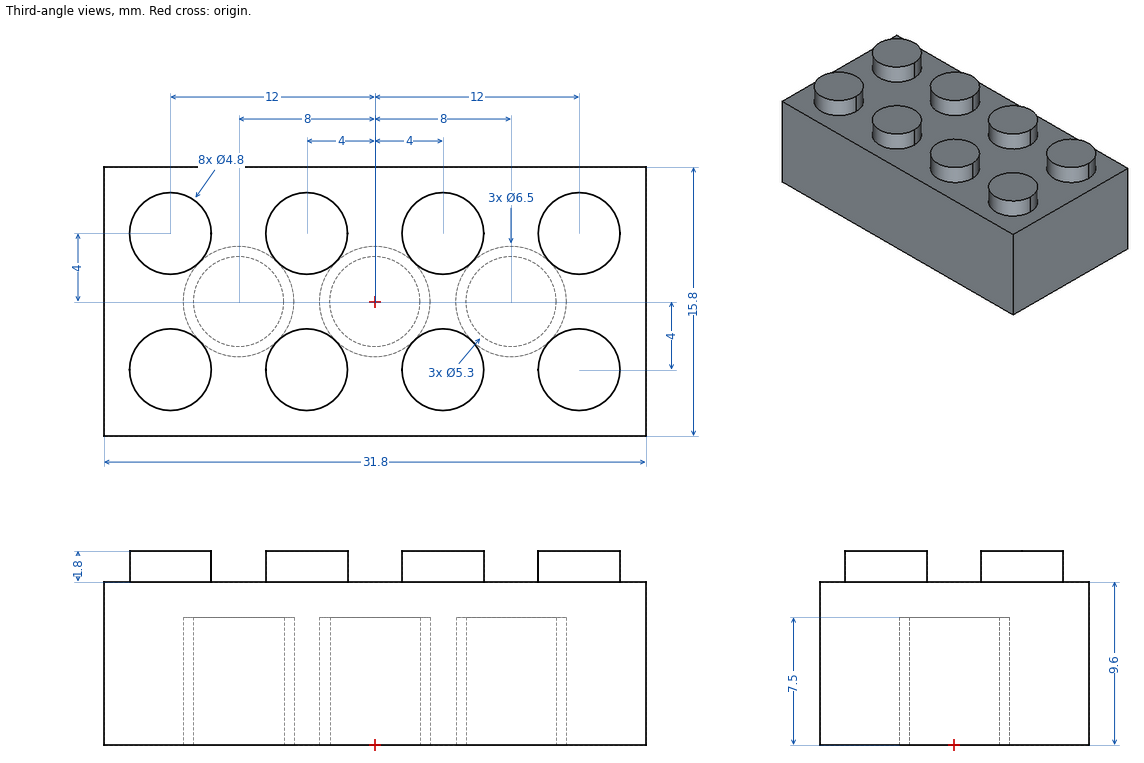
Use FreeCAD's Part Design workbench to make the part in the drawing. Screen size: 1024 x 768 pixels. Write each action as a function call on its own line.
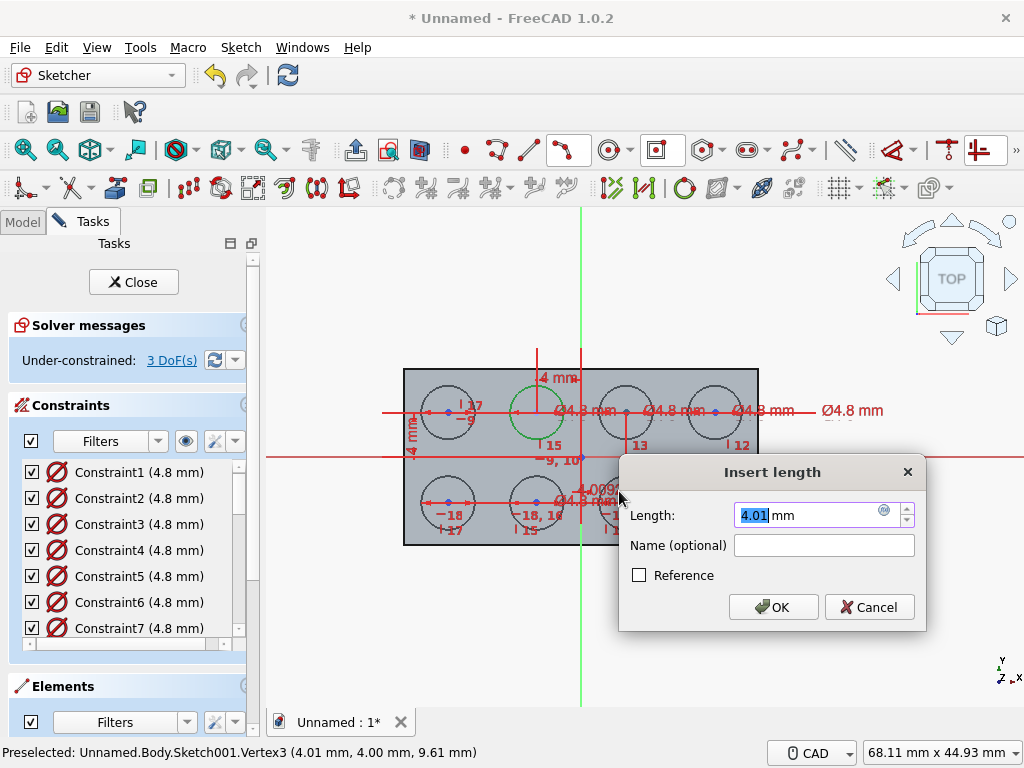
text(4)
key(Return)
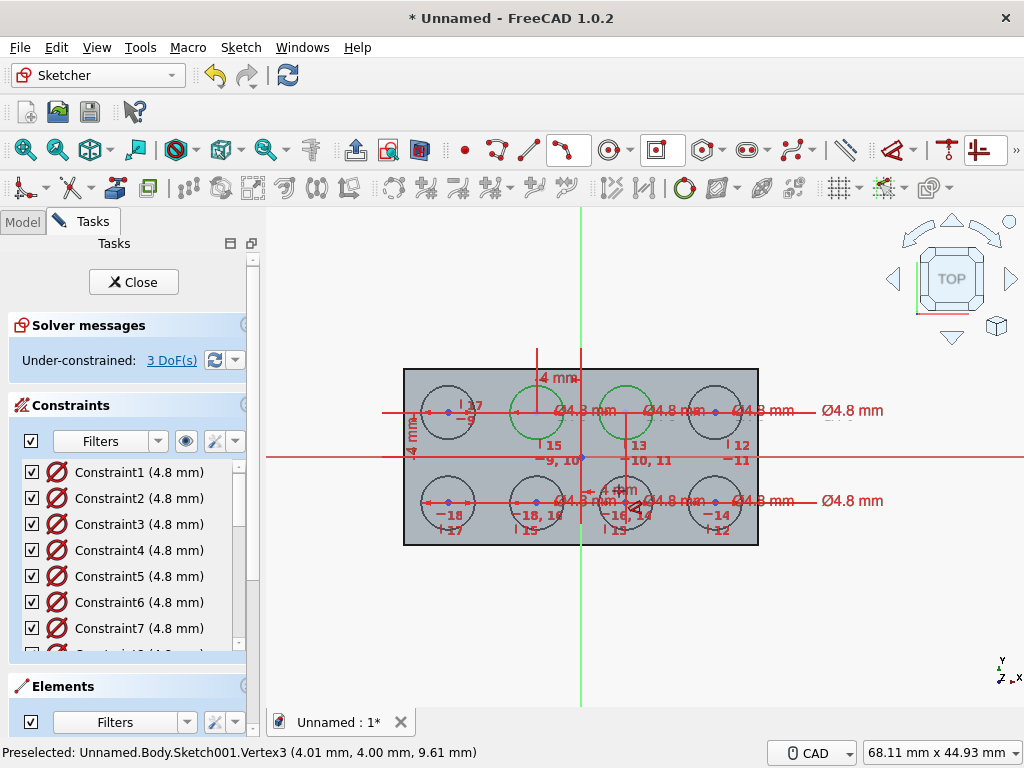
click(715, 503)
click(749, 480)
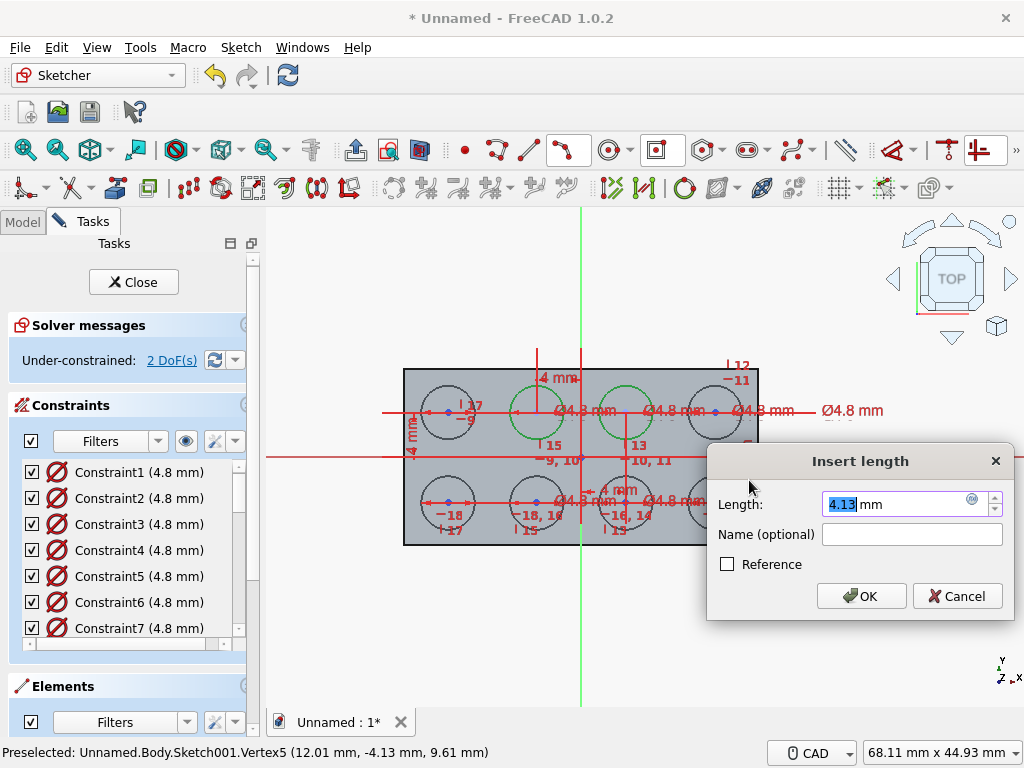
text(4)
key(Return)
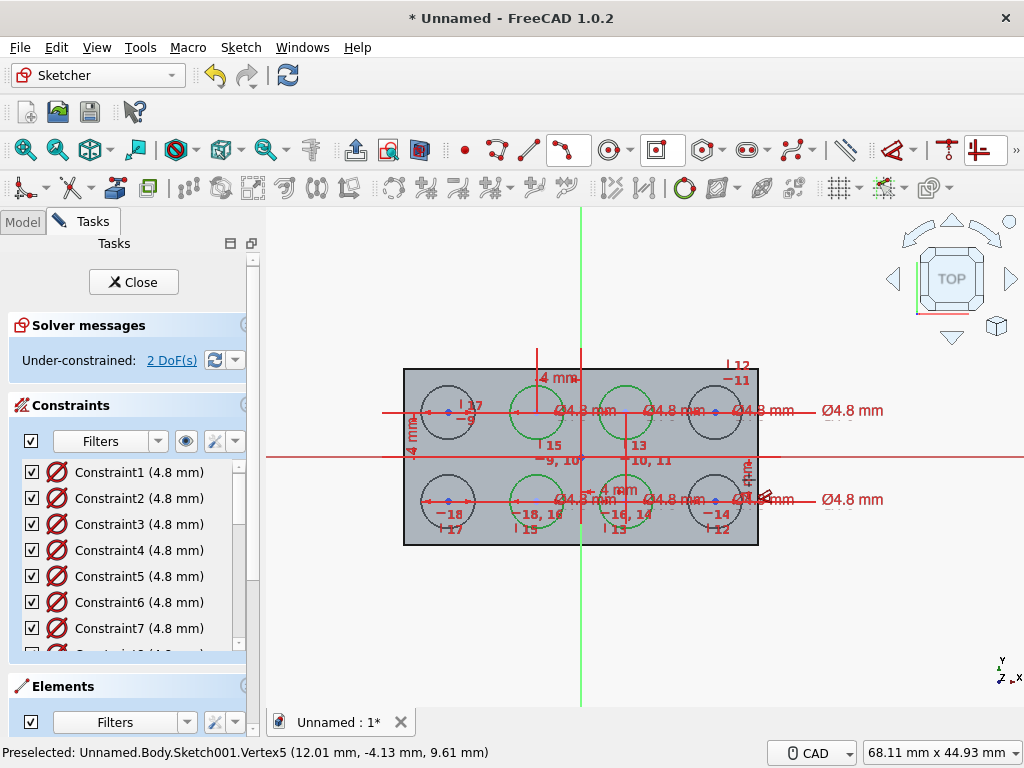
click(448, 413)
click(484, 379)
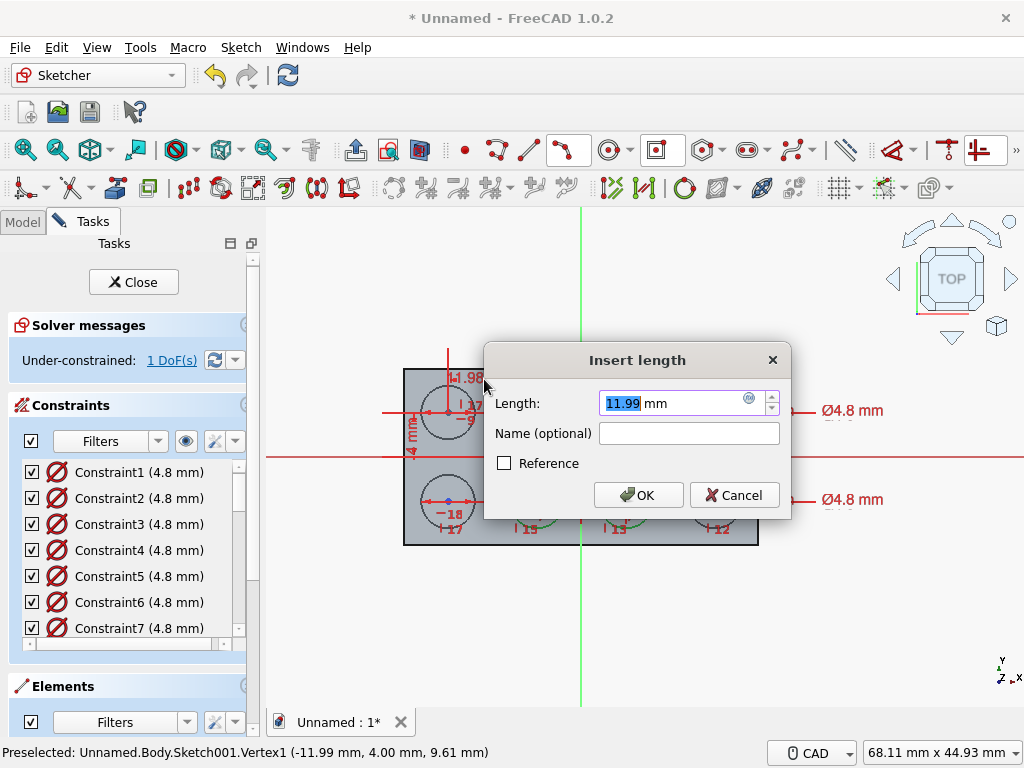
text(12)
key(Return)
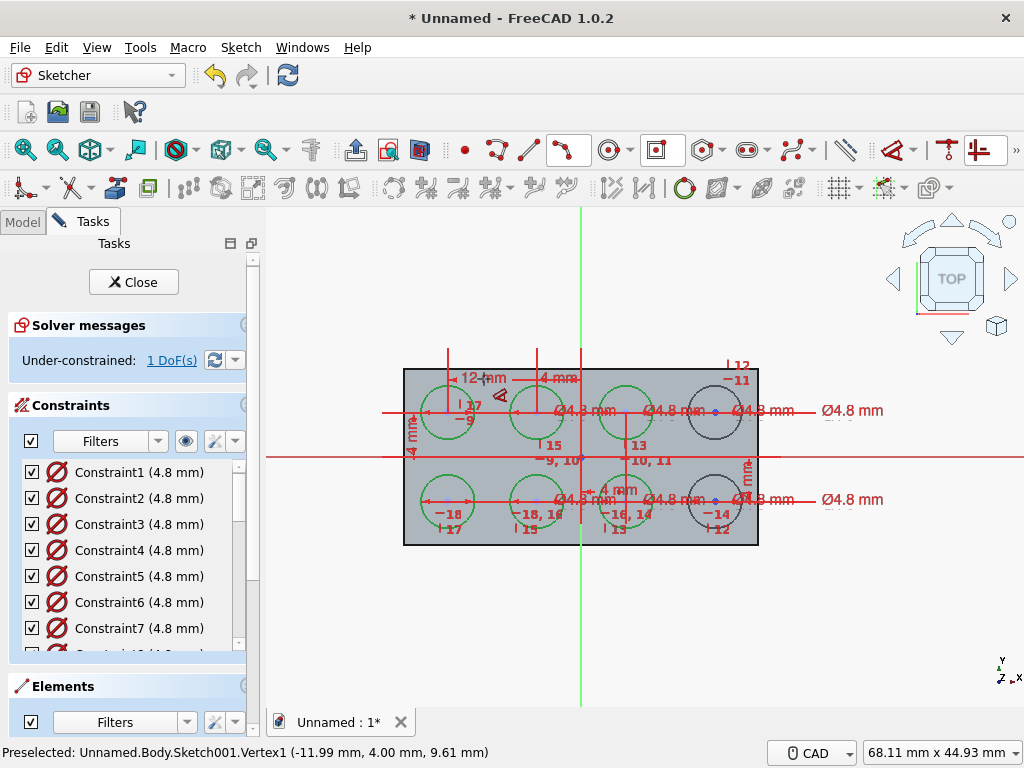
click(715, 413)
click(648, 379)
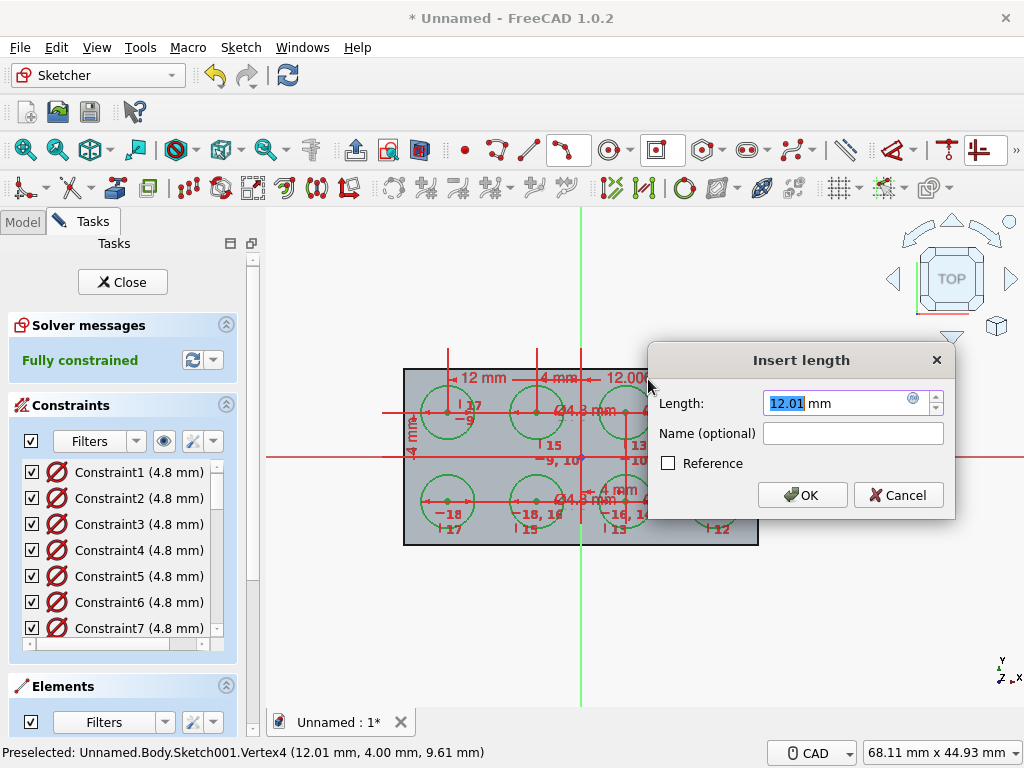
text(12)
key(Return)
key(Escape)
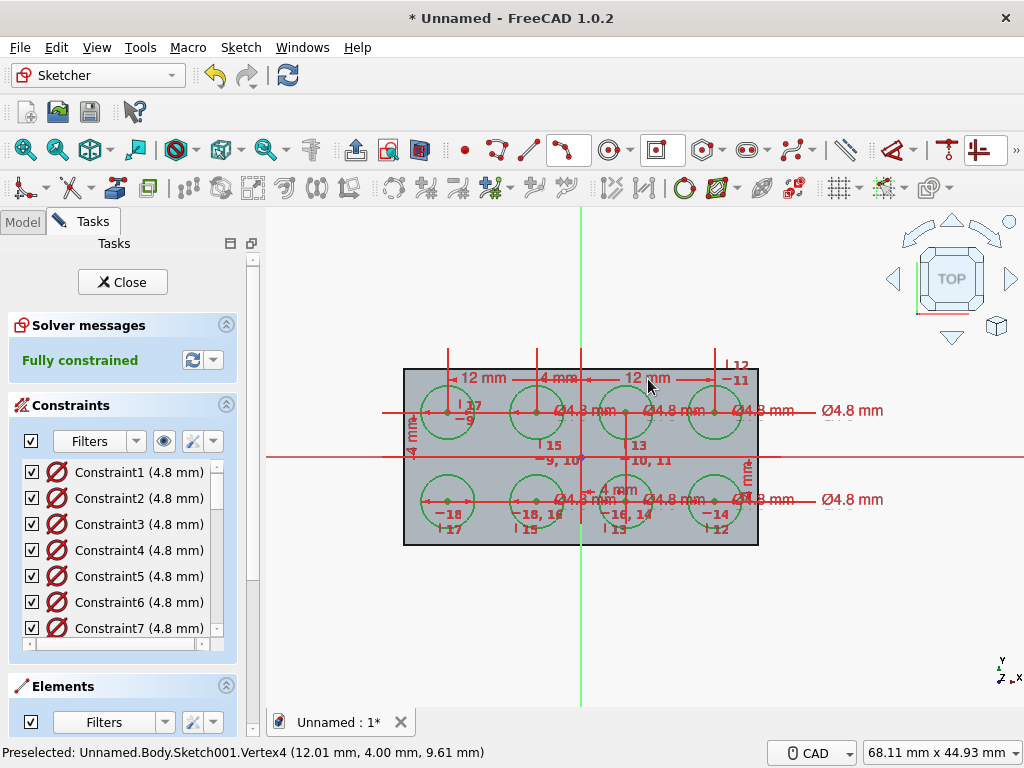
click(123, 282)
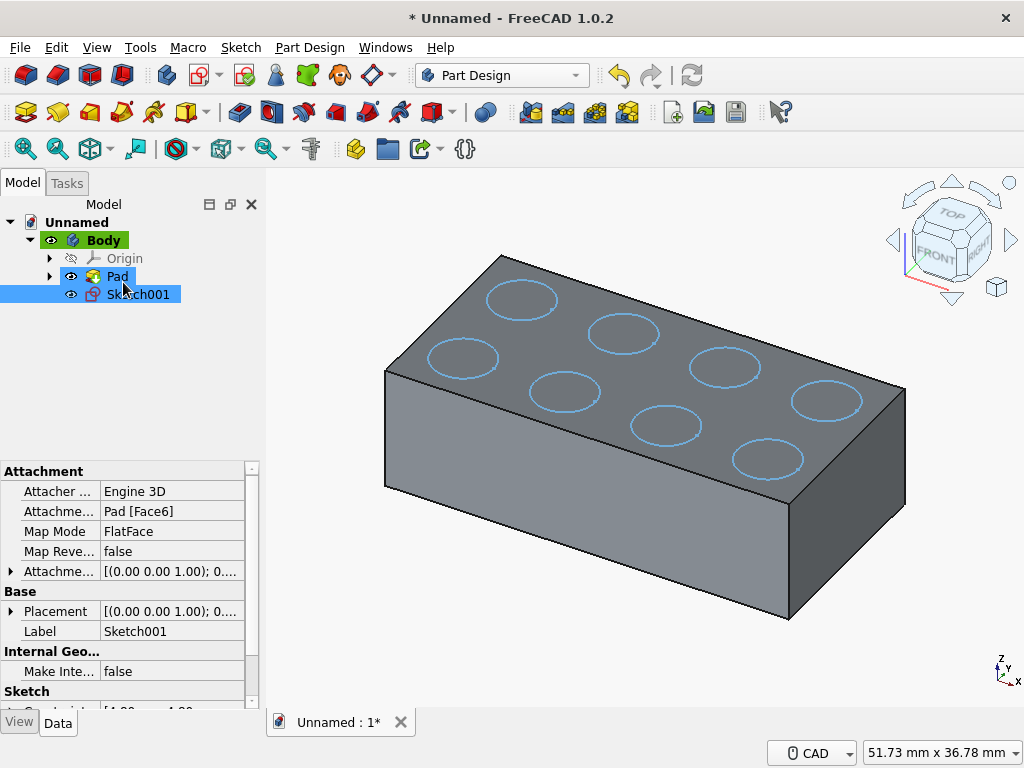
click(26, 112)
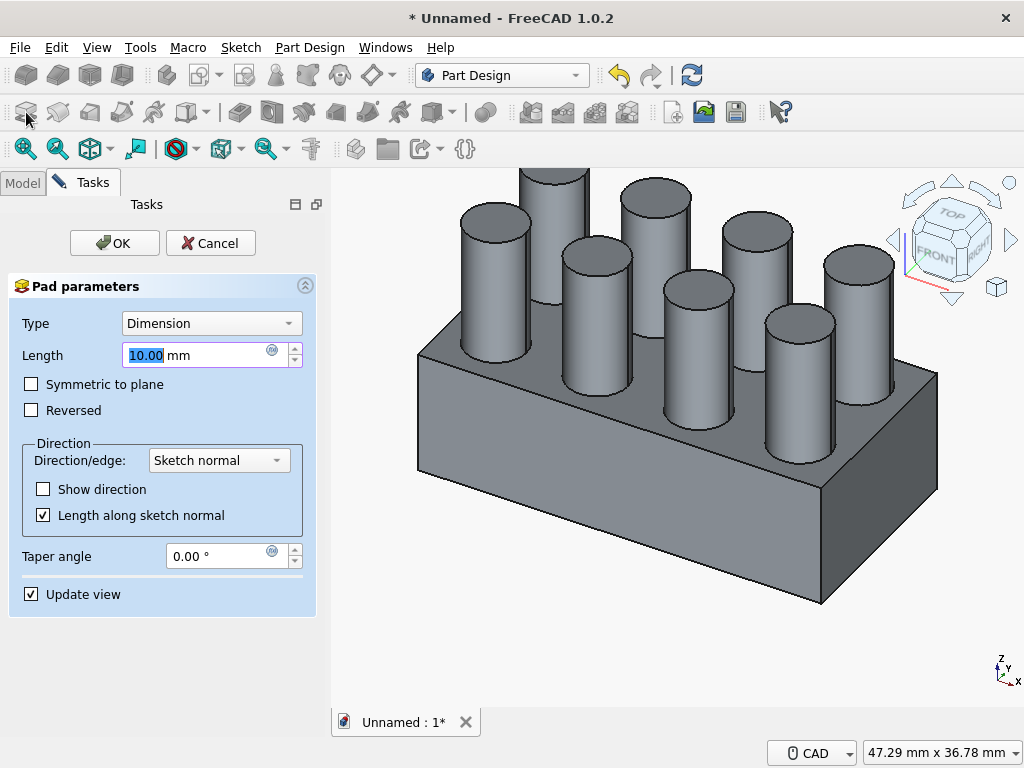
text(1.8)
key(Tab)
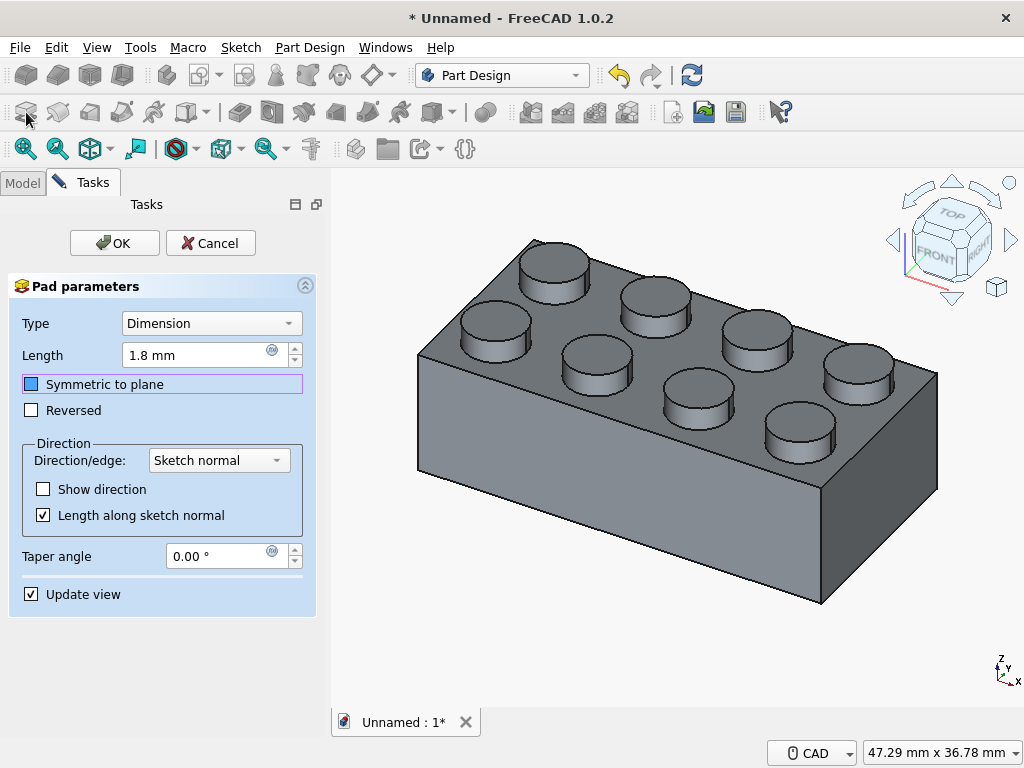
click(115, 243)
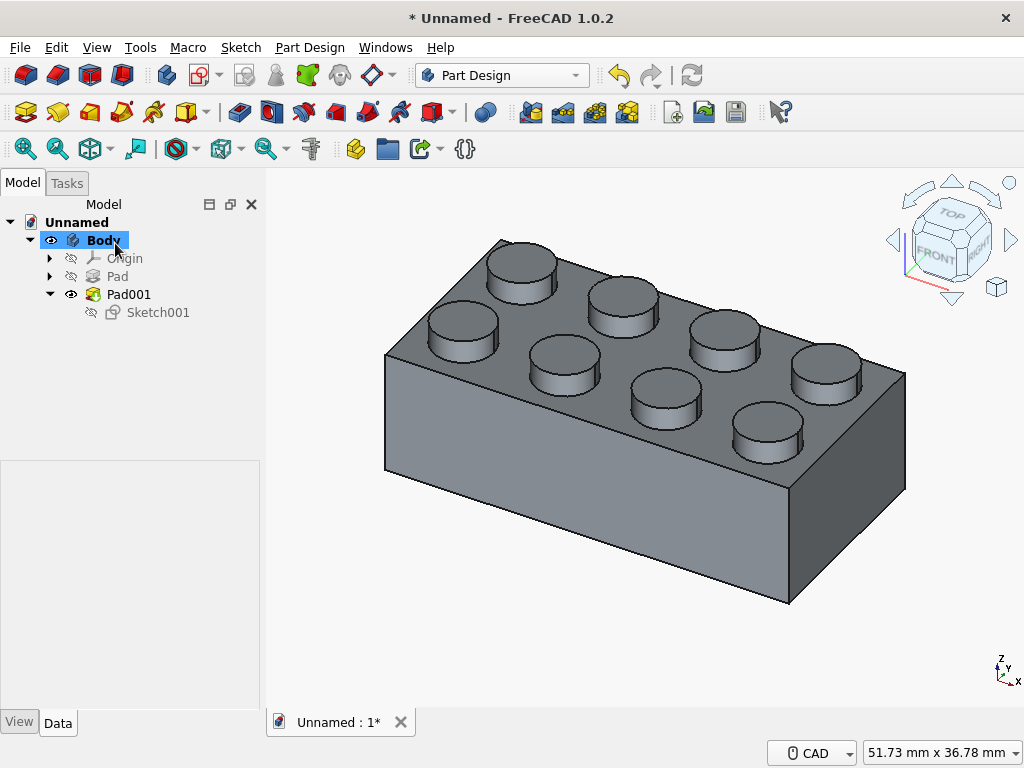
key(5)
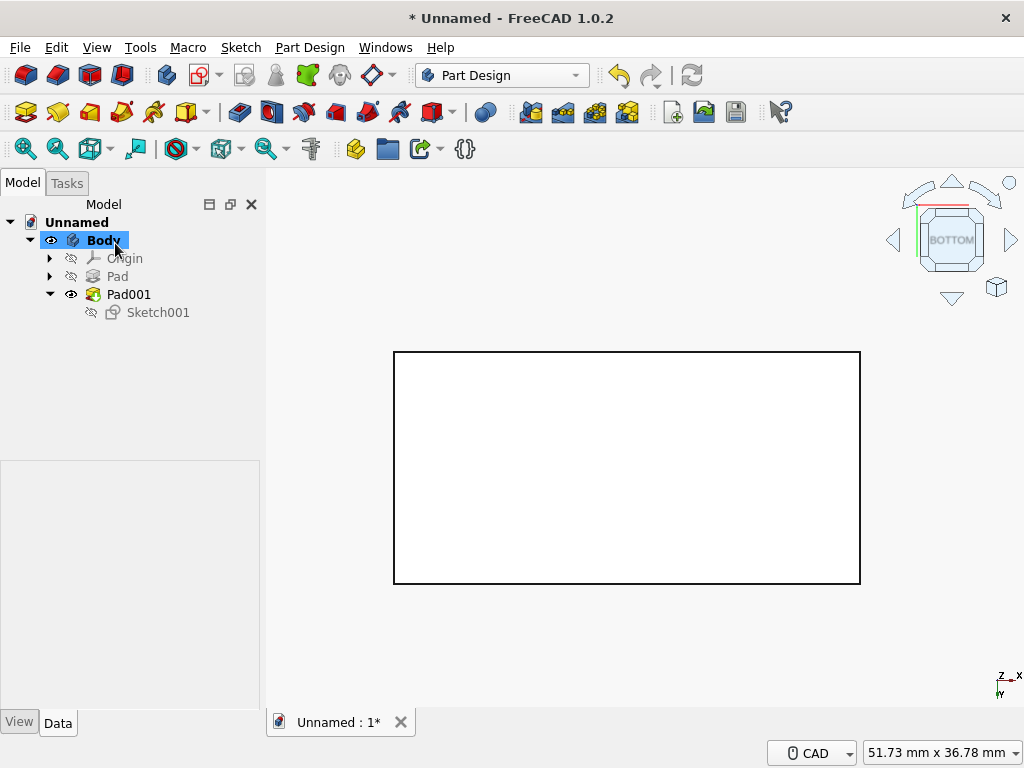
click(694, 467)